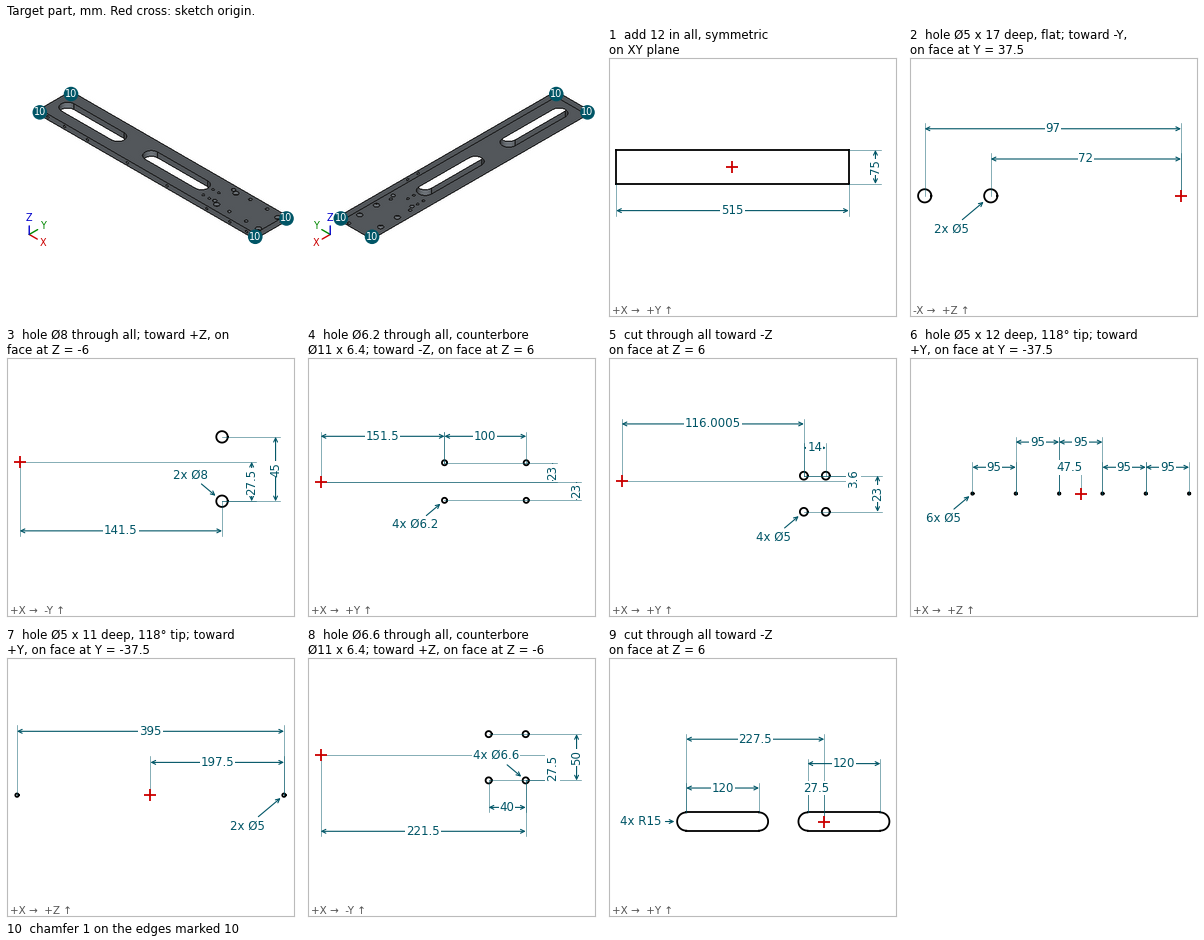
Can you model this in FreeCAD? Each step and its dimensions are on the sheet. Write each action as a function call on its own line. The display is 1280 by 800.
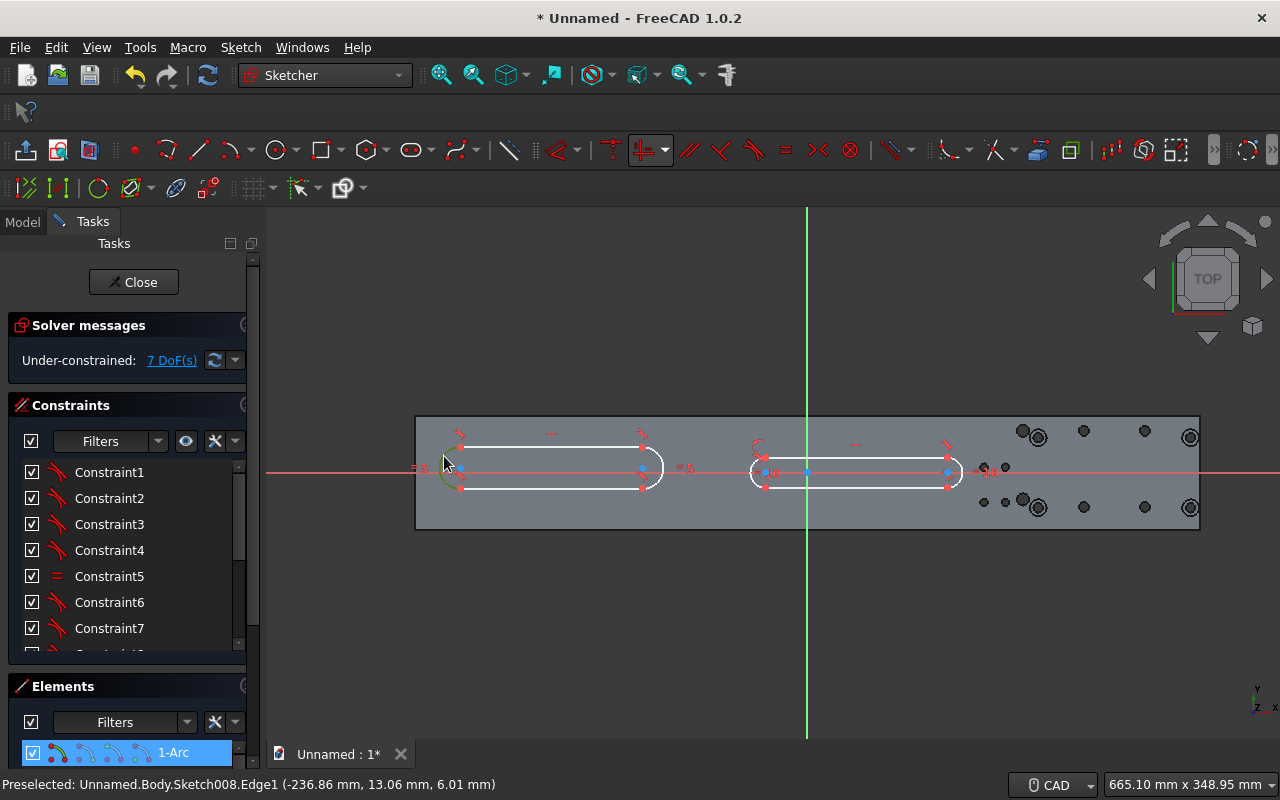
click(750, 473)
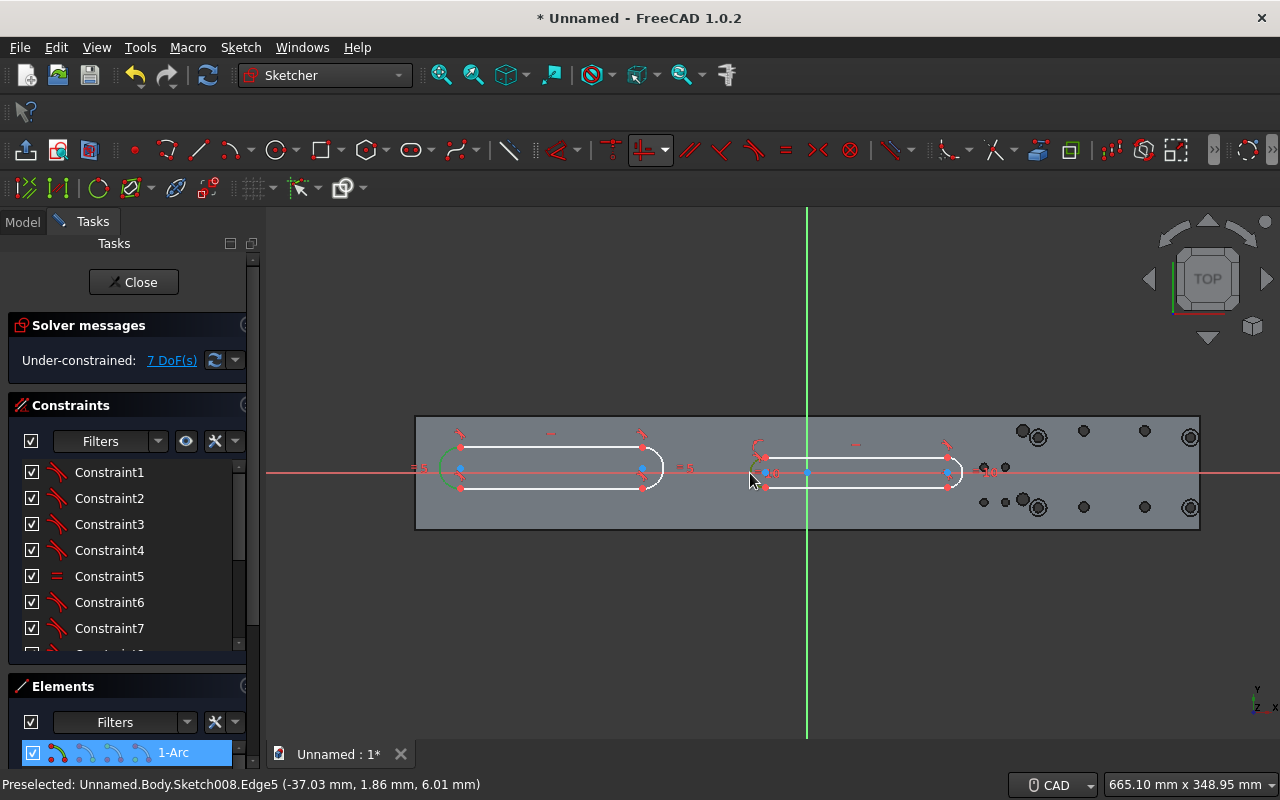
click(786, 150)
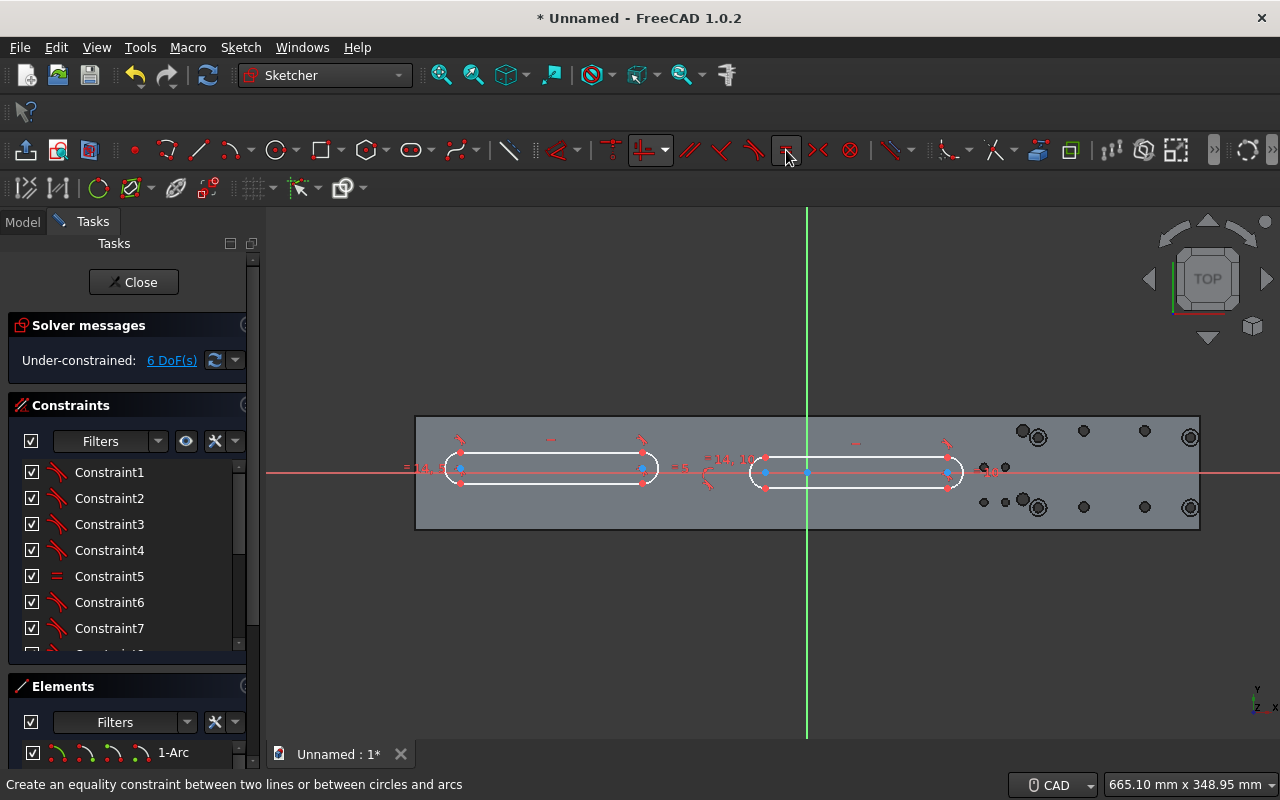
click(460, 468)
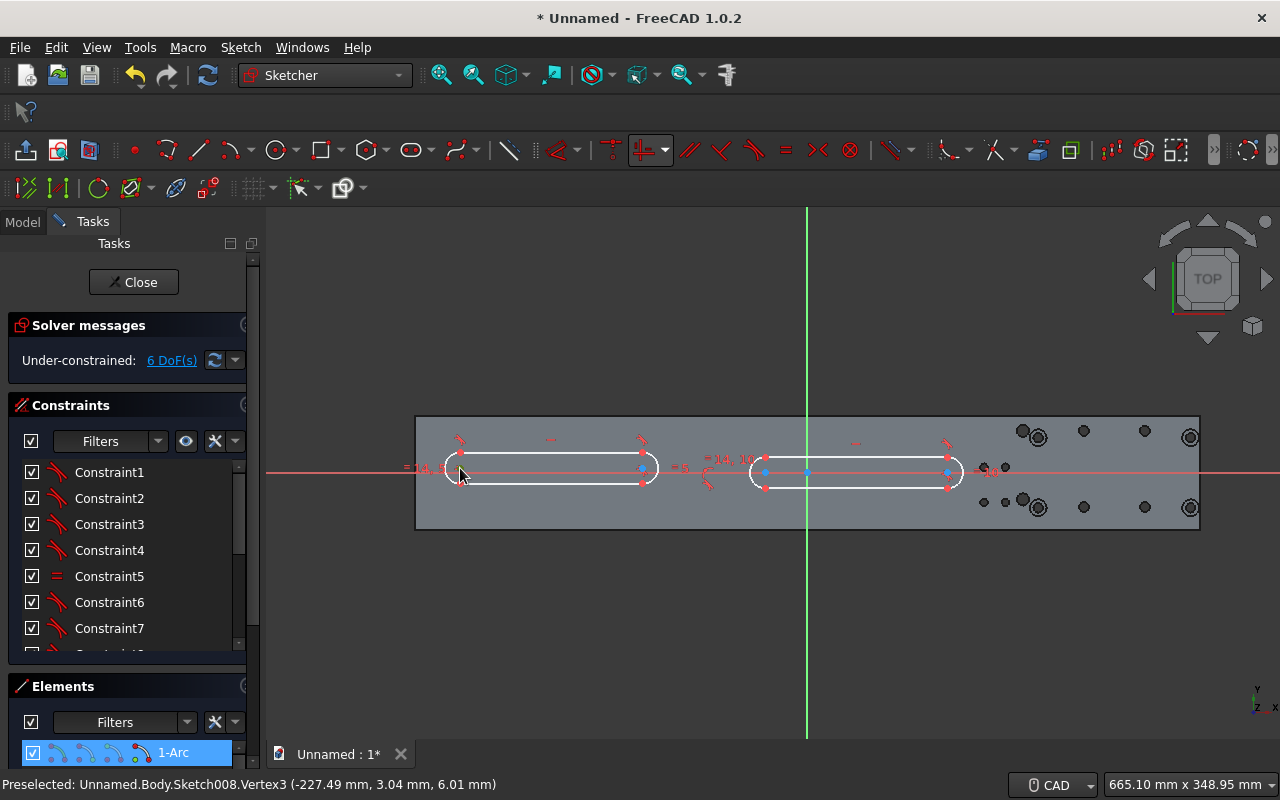
click(353, 473)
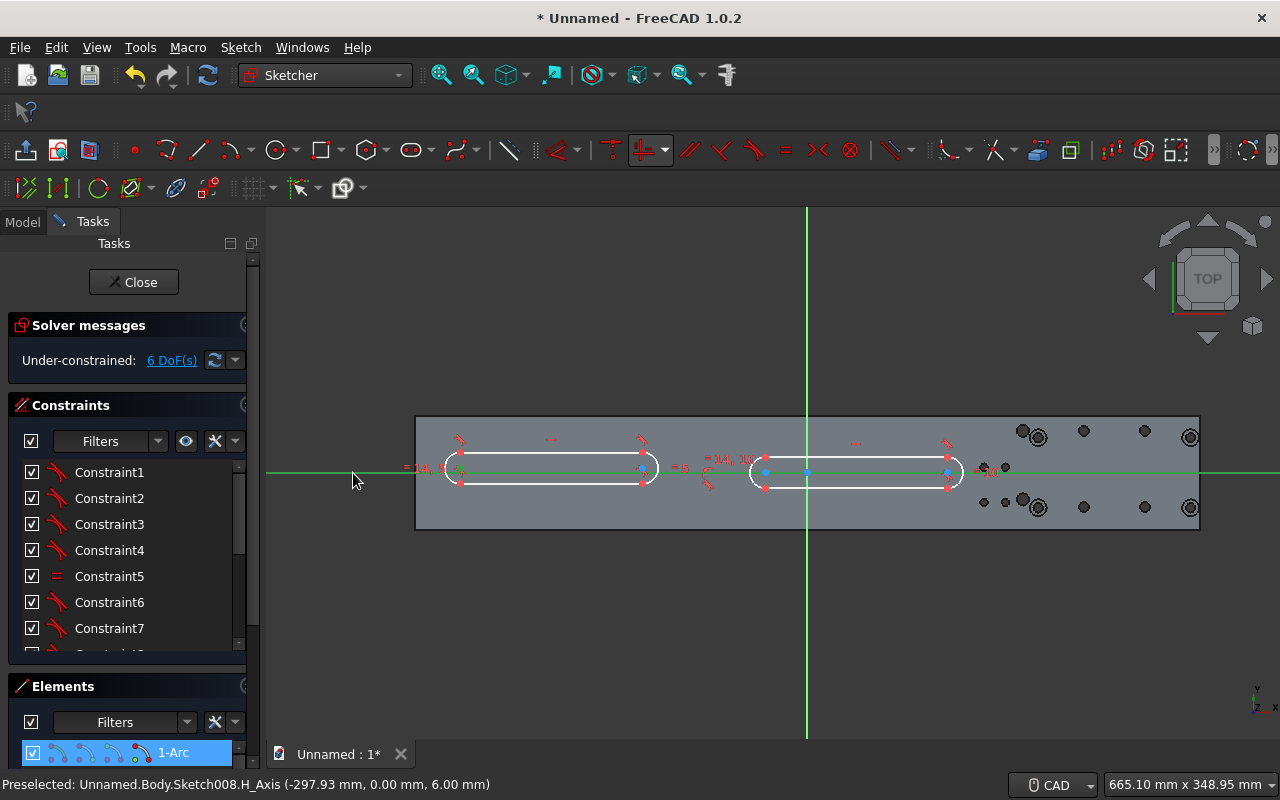
key(c)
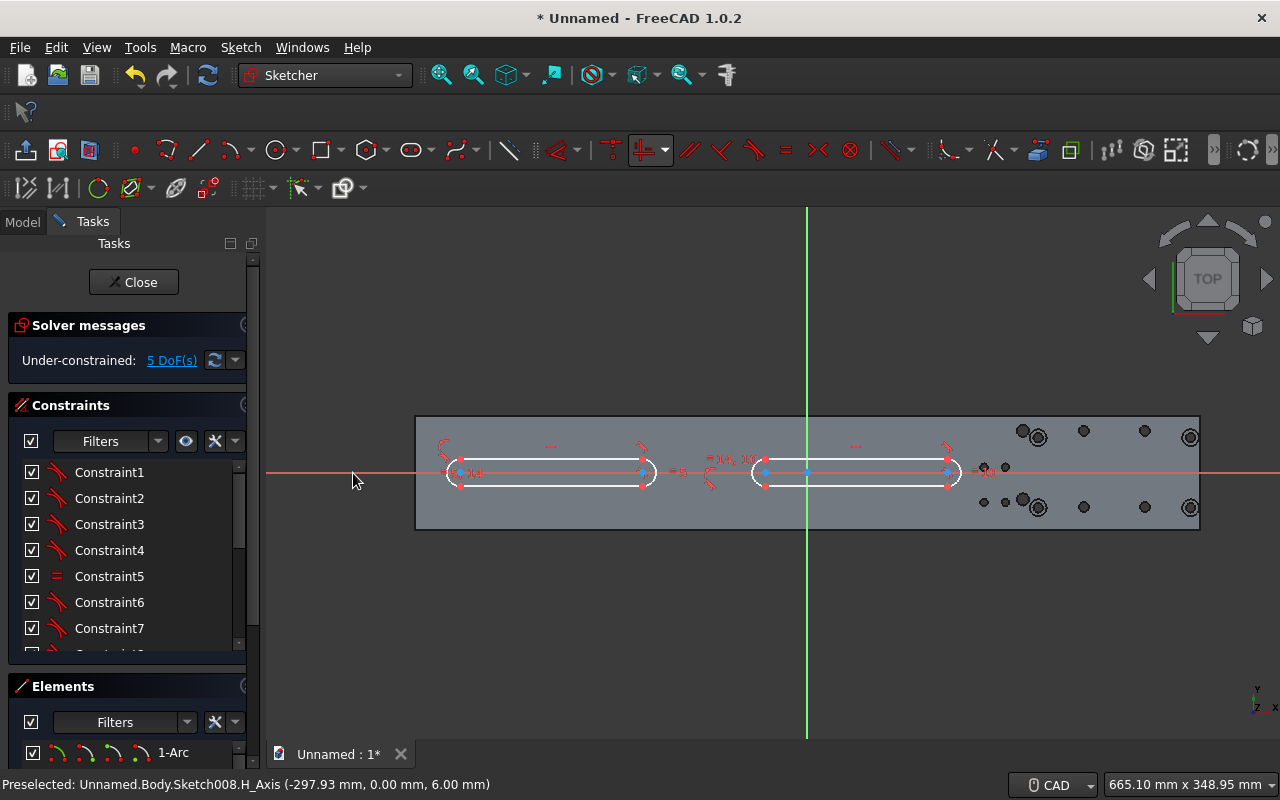
key(d)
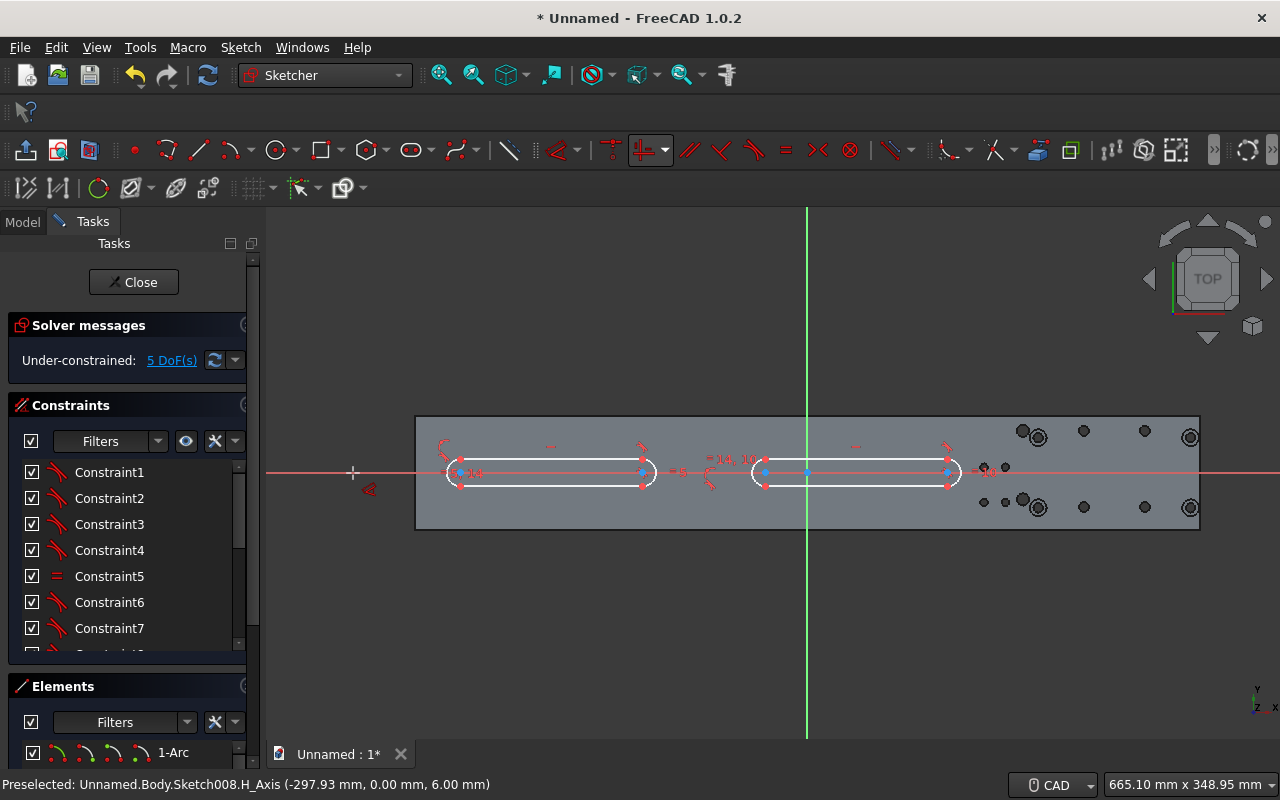
scroll(447, 473, up, 3)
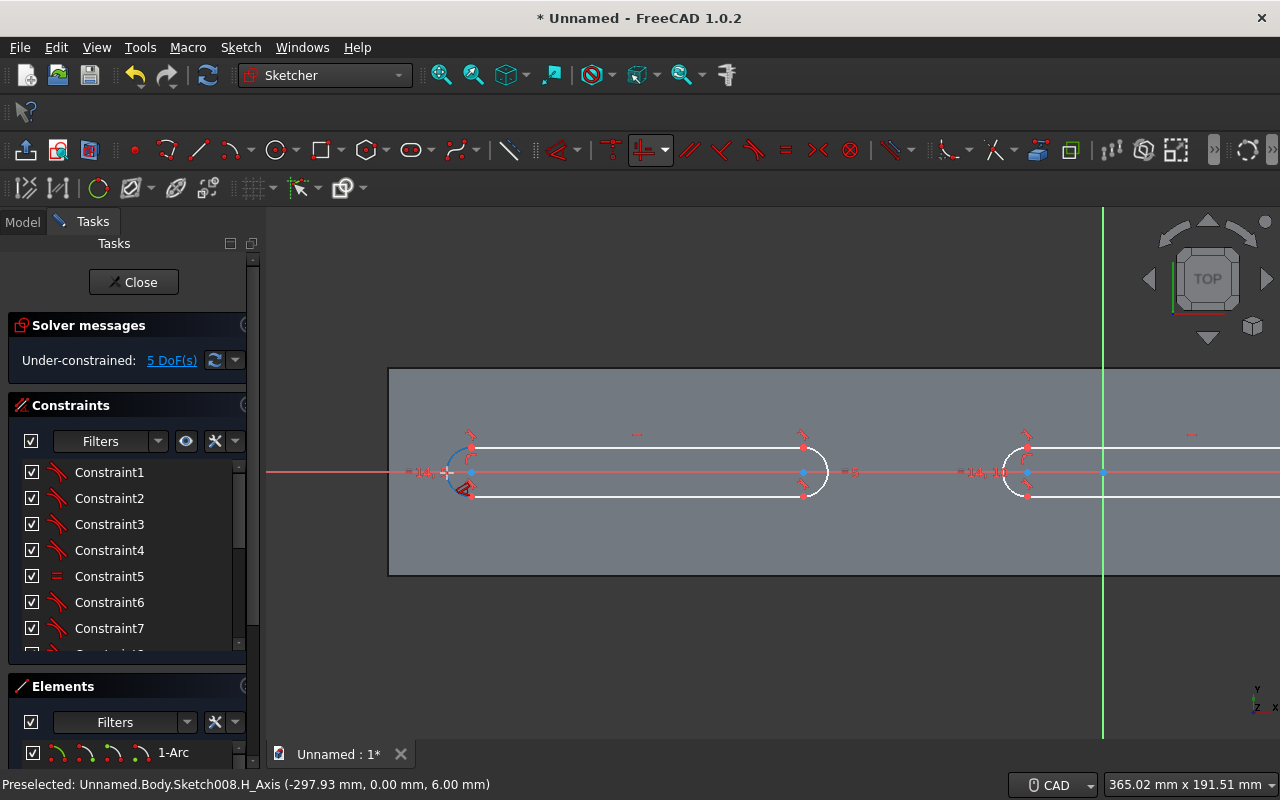
click(447, 472)
click(422, 445)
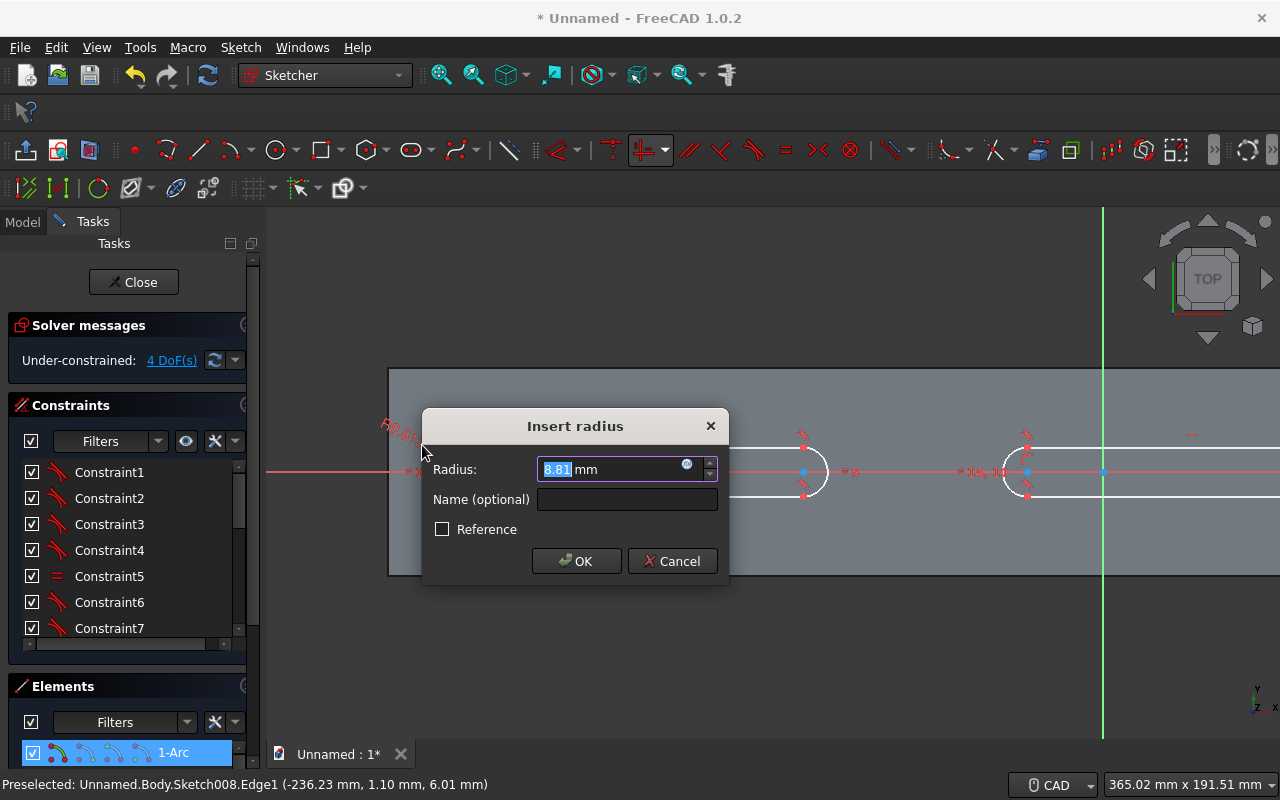
text(15)
key(Return)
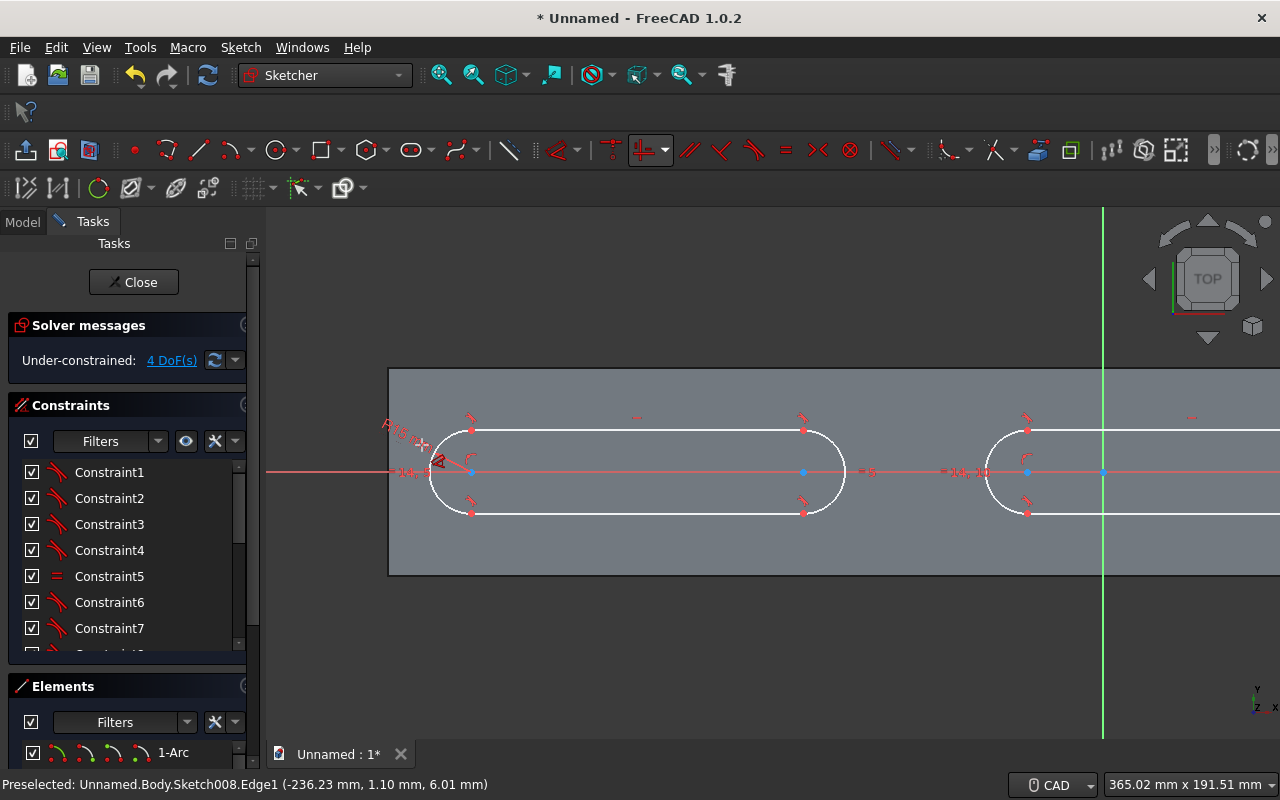
click(571, 430)
click(637, 396)